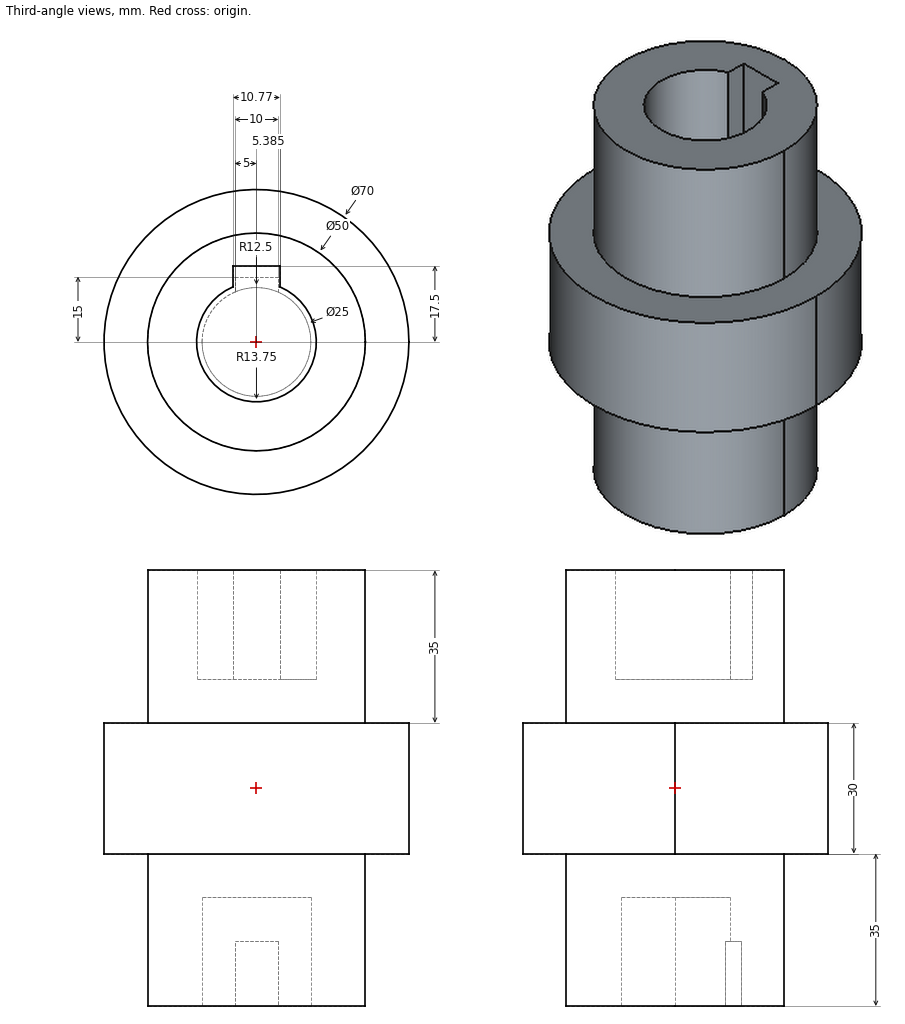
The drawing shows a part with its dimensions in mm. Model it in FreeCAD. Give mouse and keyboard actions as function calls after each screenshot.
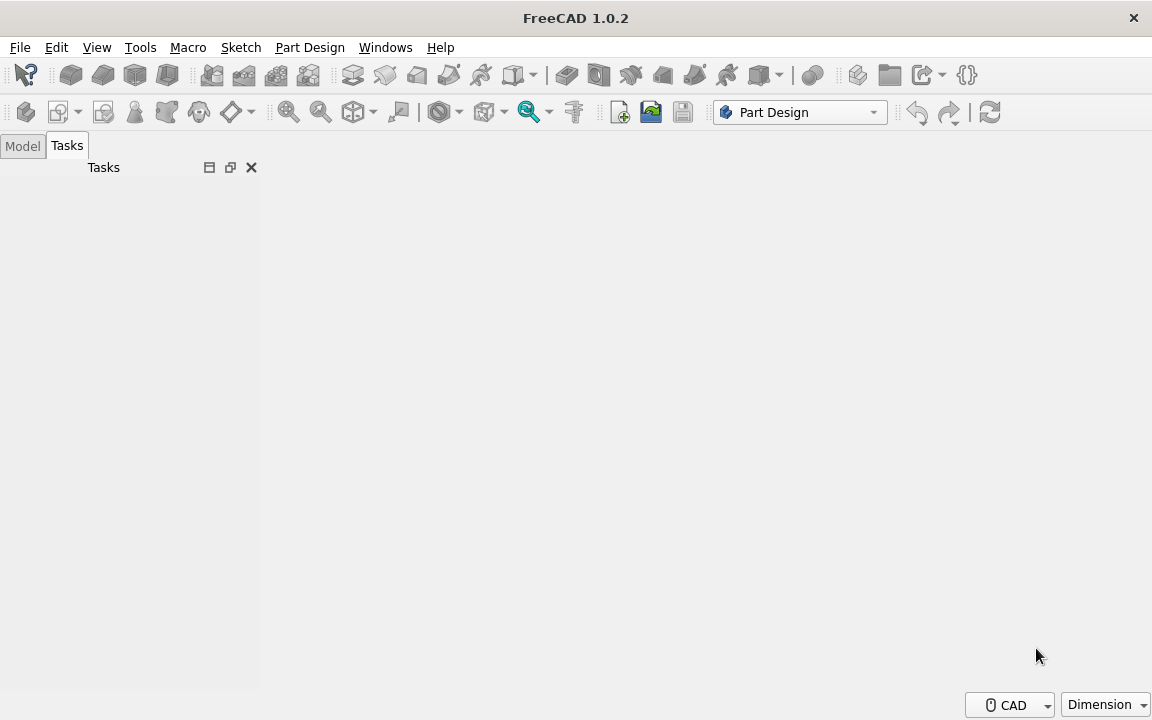
key(ctrl+n)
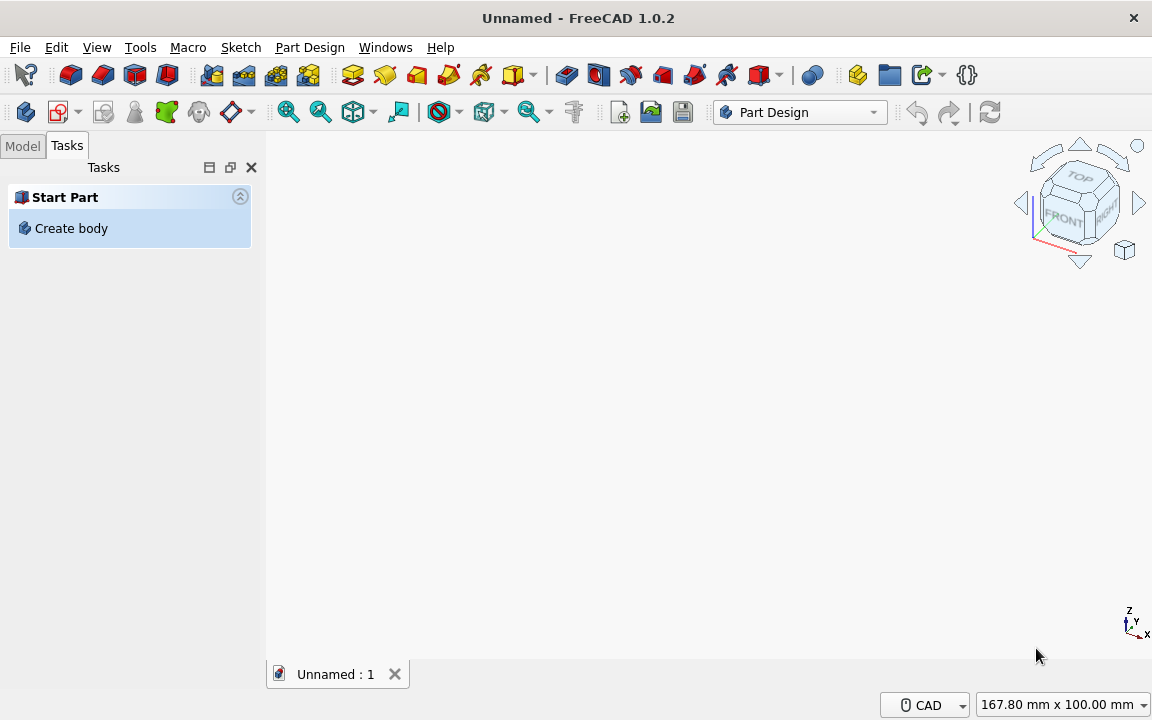
click(58, 112)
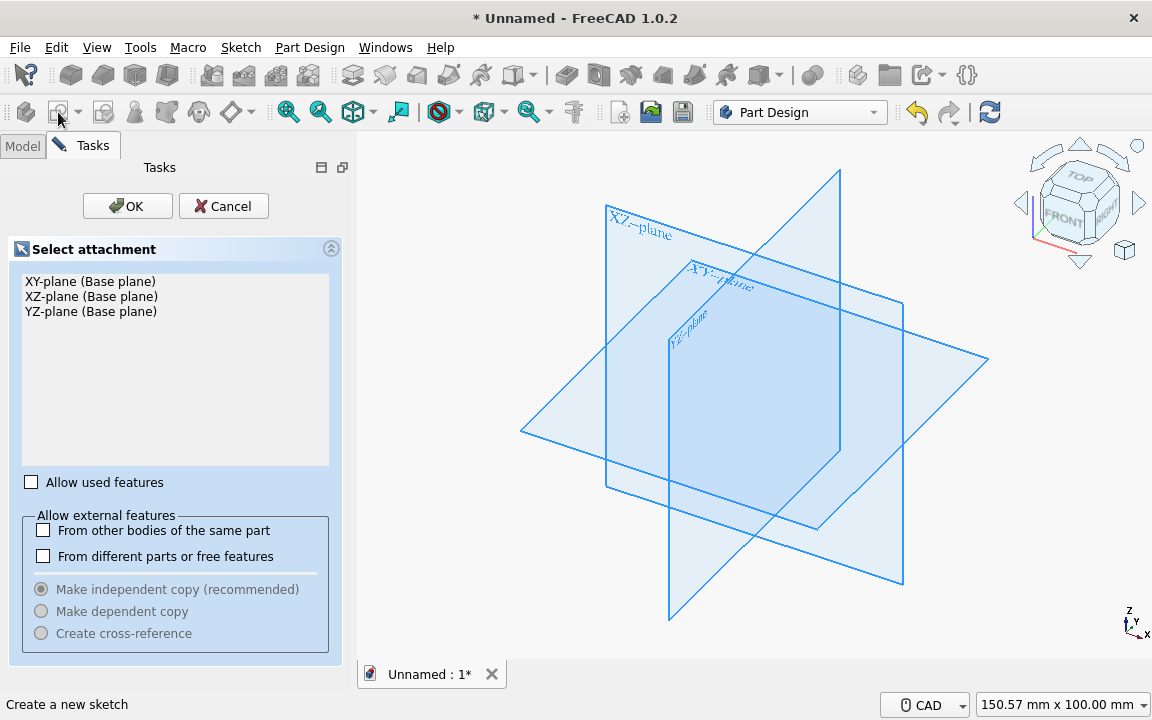
click(82, 282)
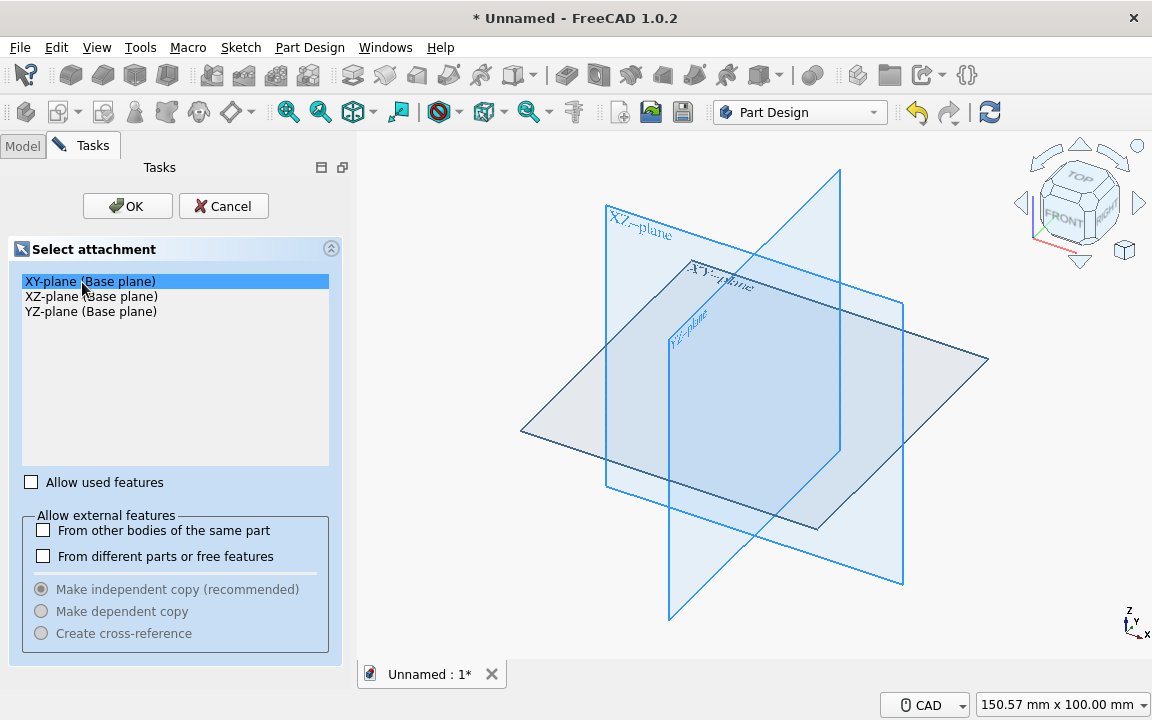
click(128, 206)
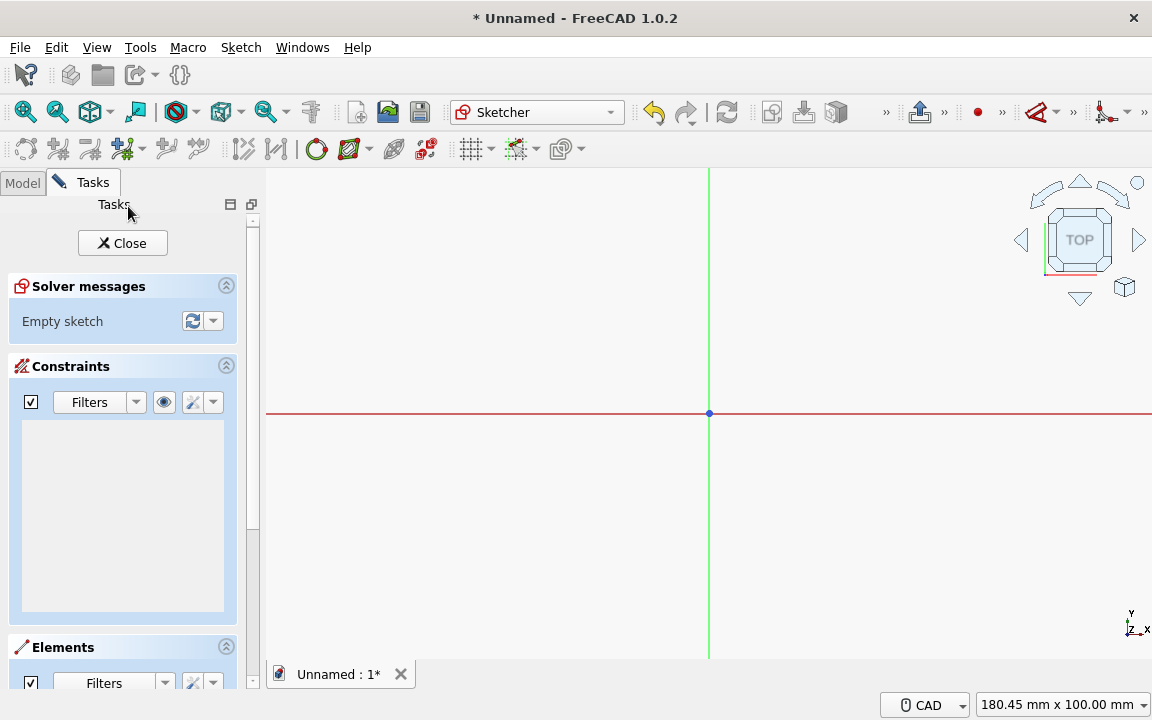
key(g)
key(c)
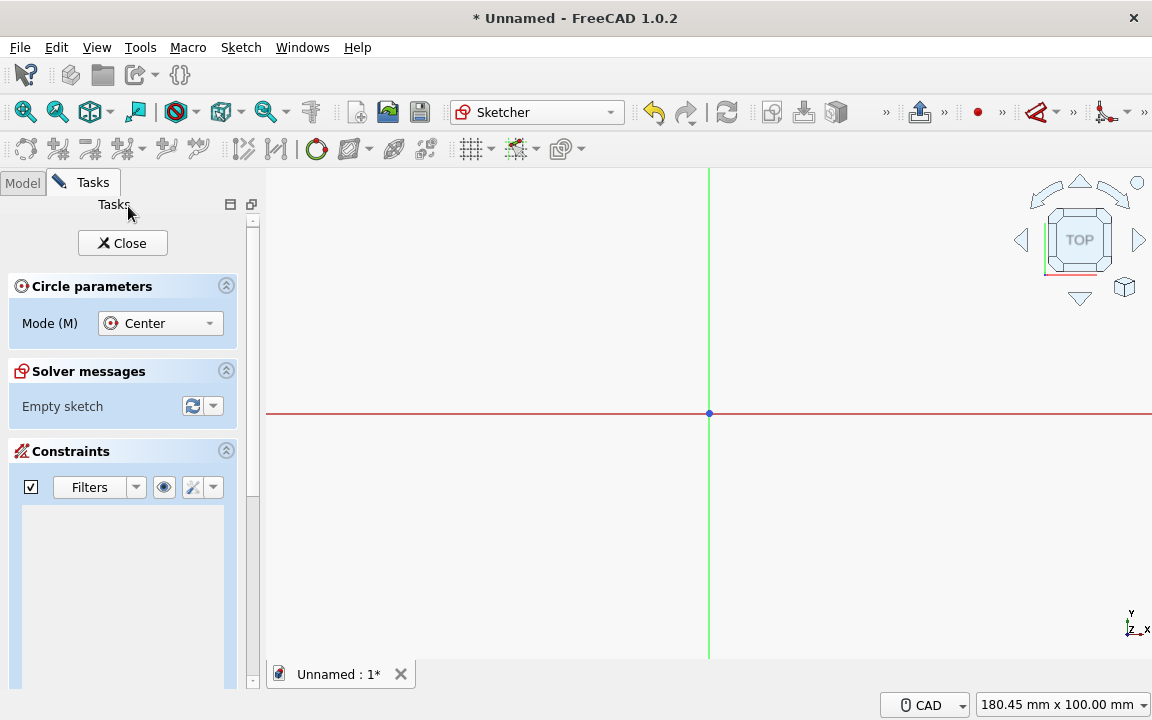
click(709, 414)
move(831, 292)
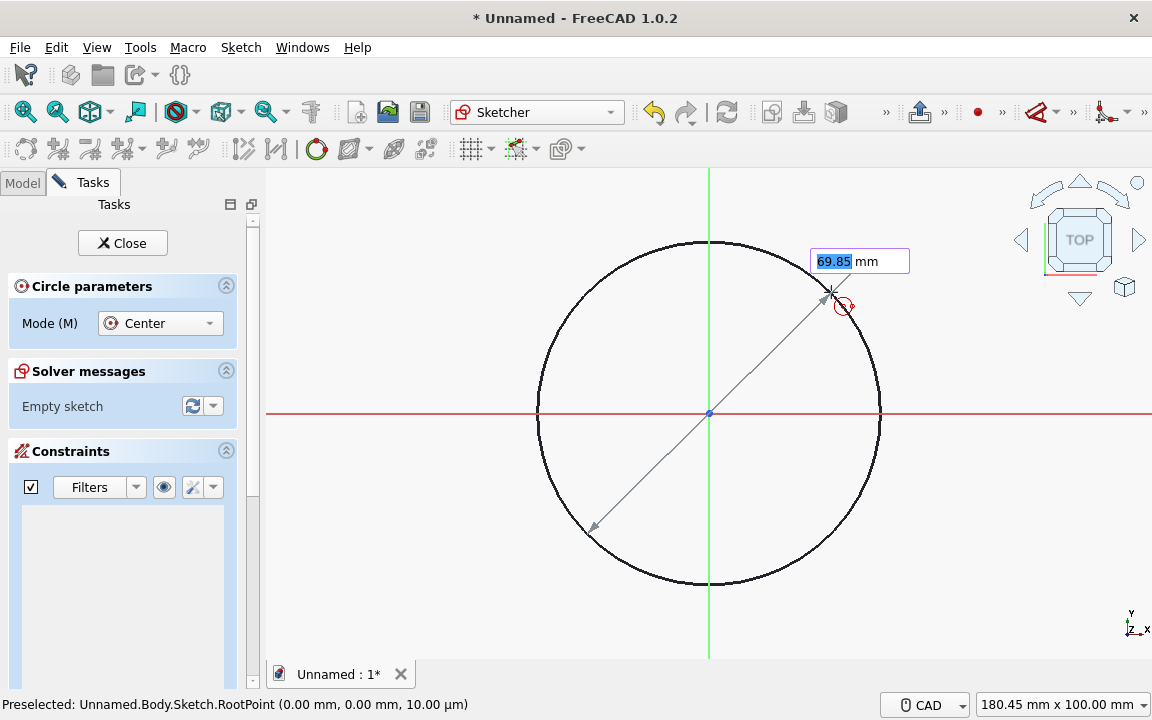
text(70)
key(Return)
key(Escape)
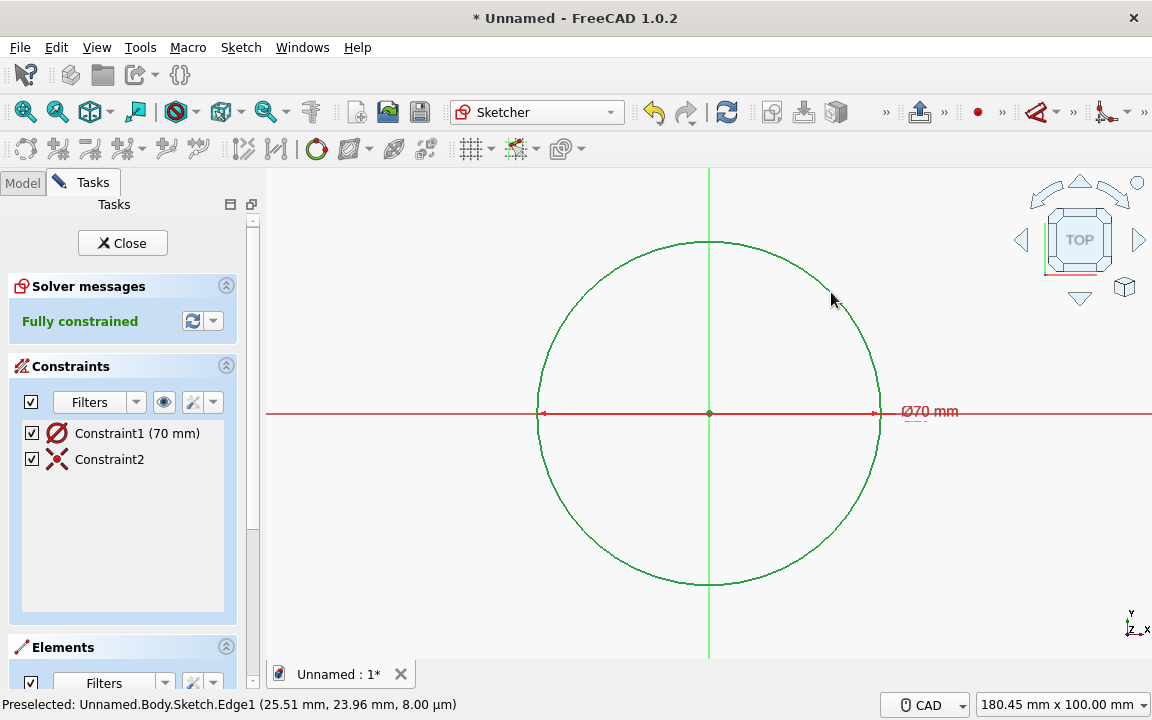
click(123, 243)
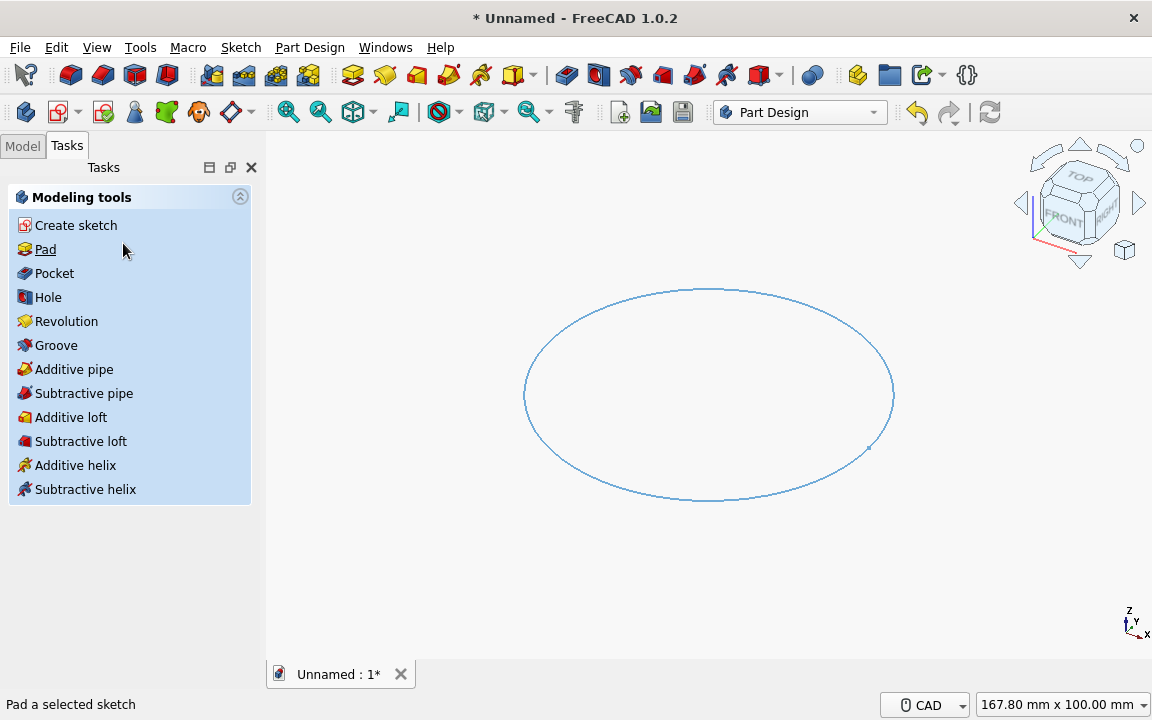
click(354, 76)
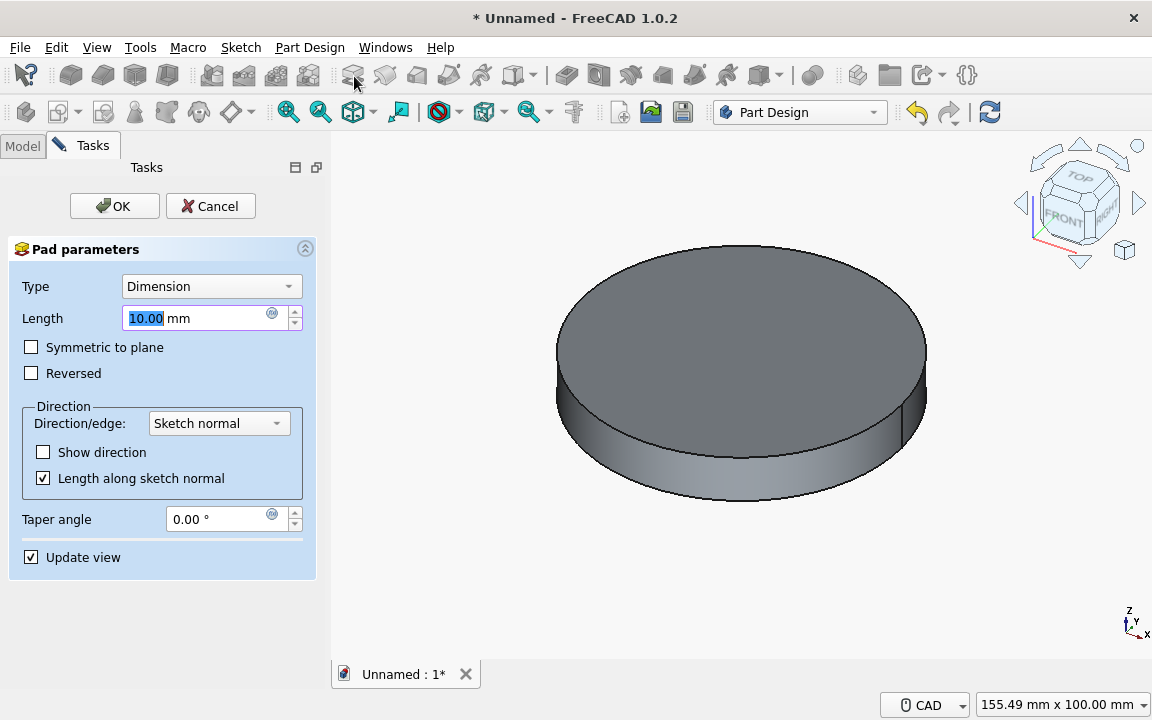
text(30)
key(Tab)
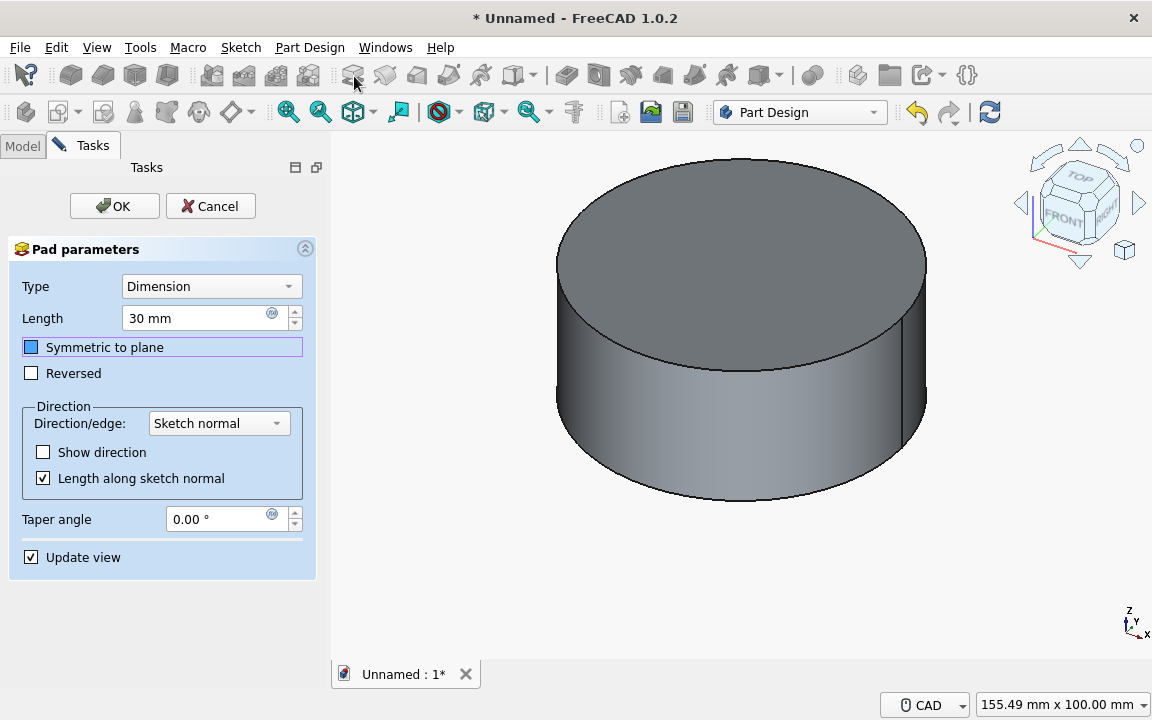
click(30, 347)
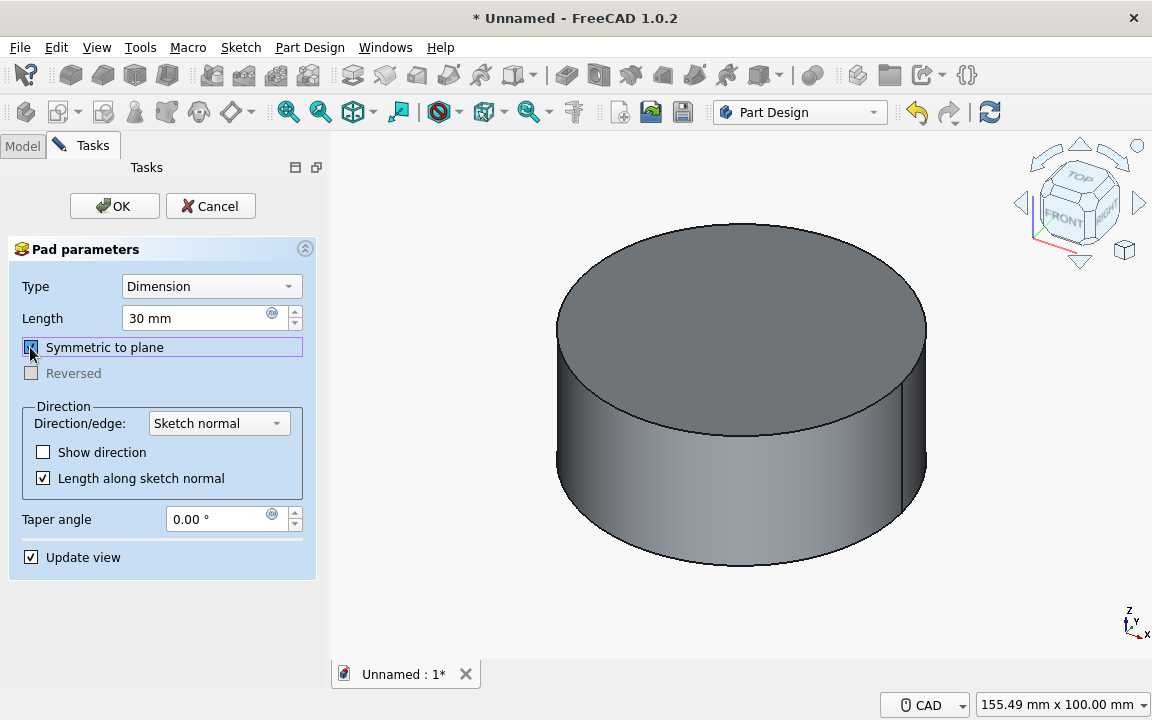
click(115, 206)